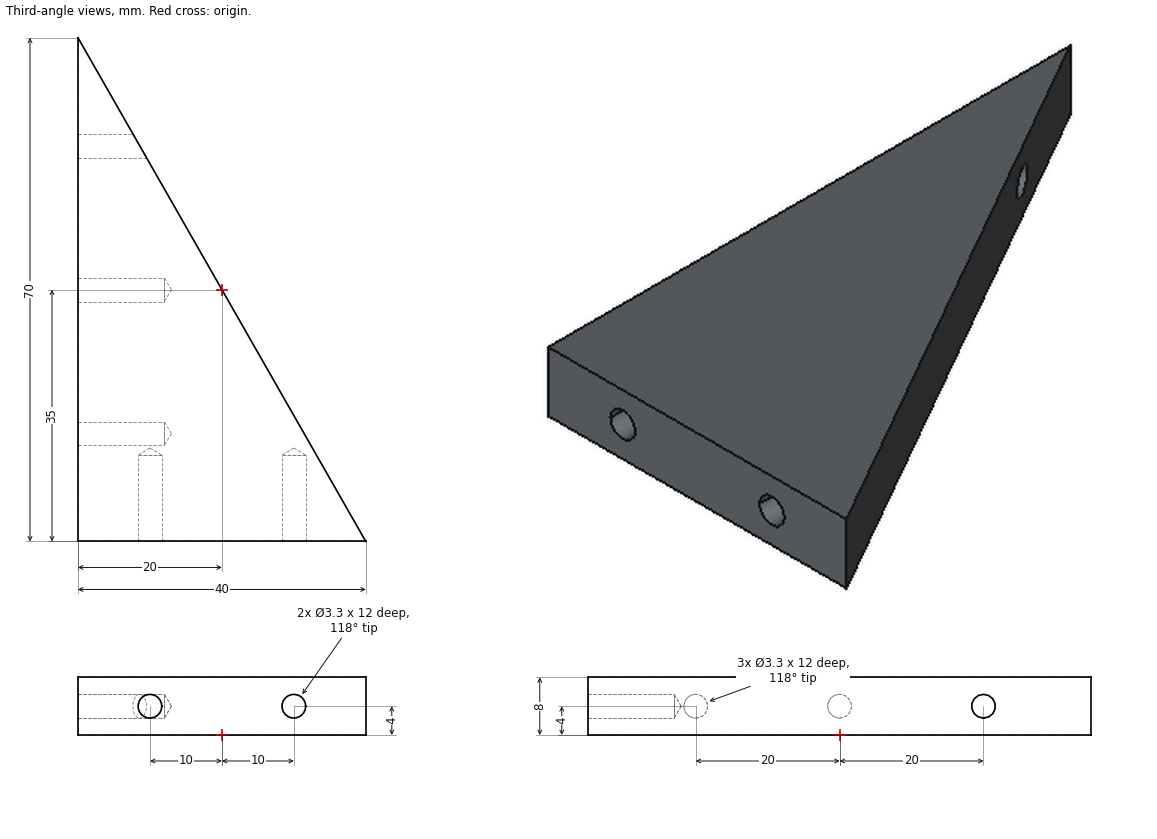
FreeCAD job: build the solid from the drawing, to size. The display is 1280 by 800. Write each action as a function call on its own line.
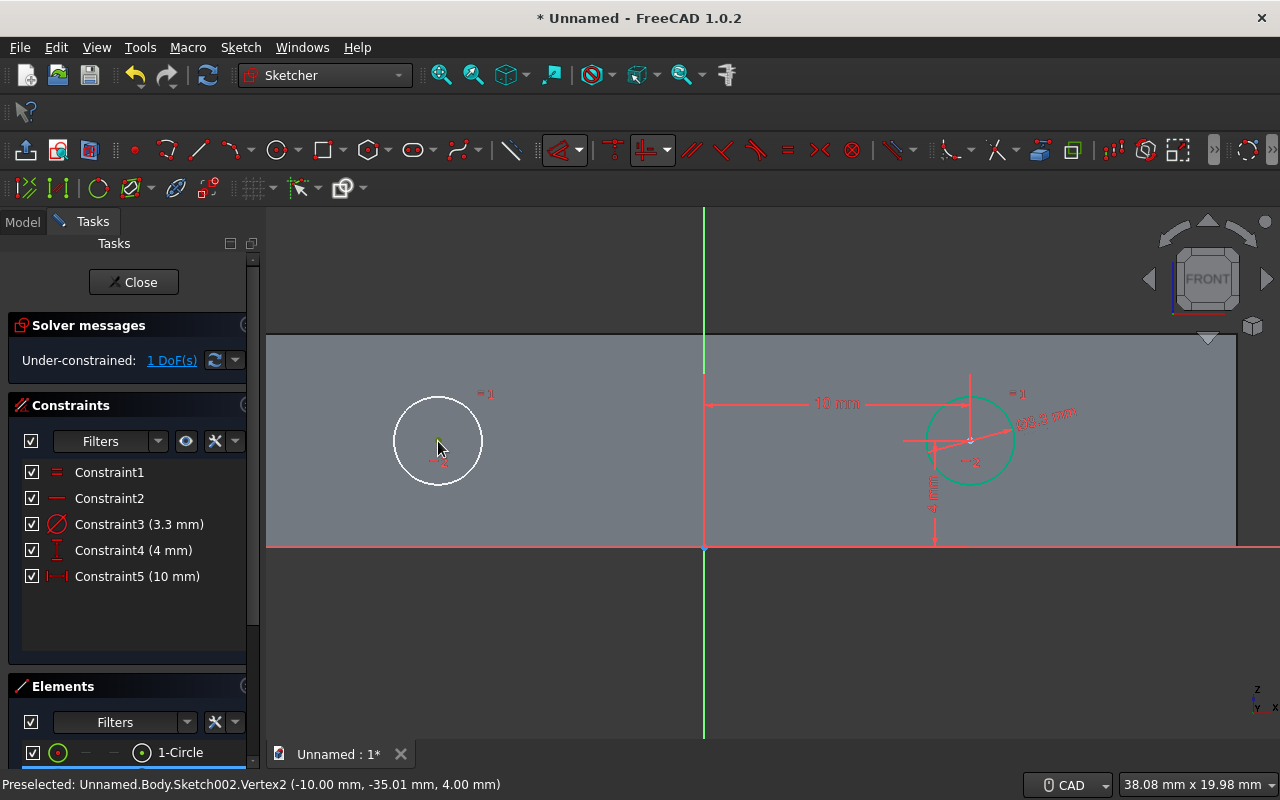
click(582, 150)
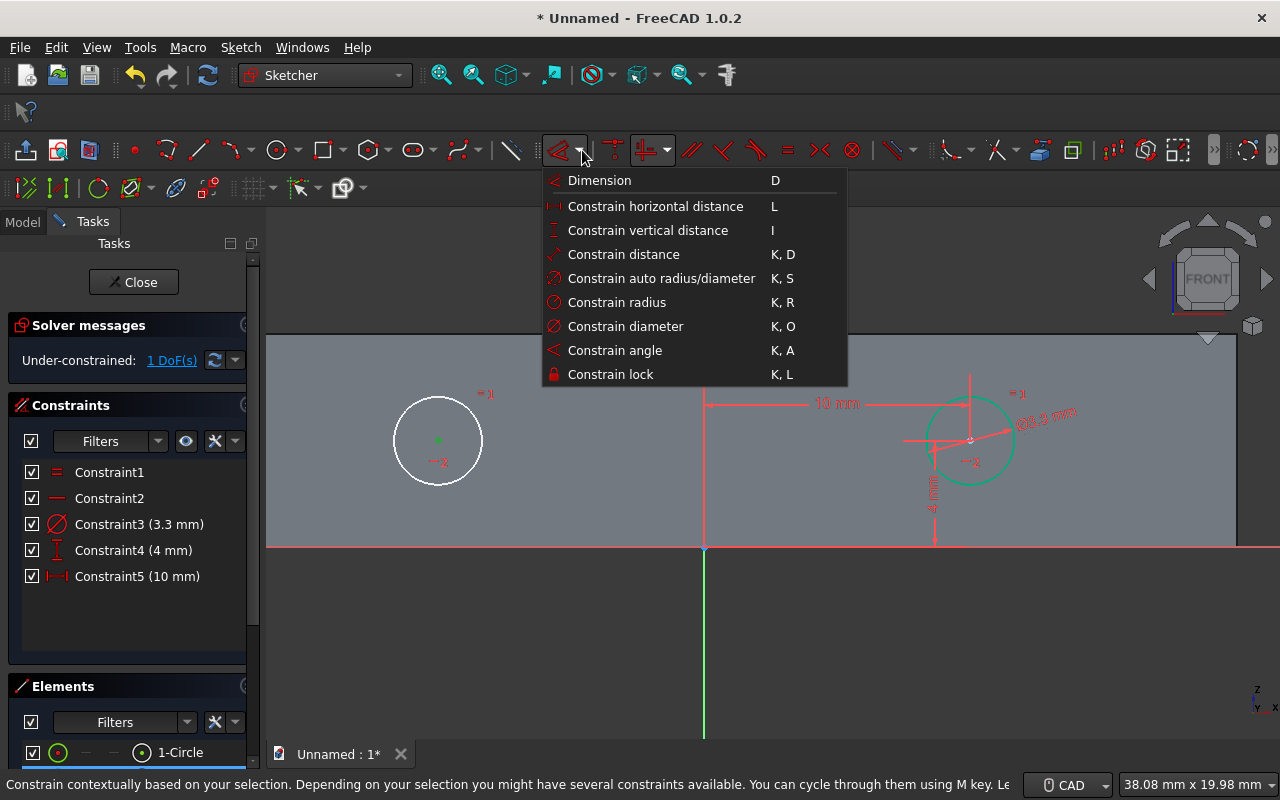
click(695, 206)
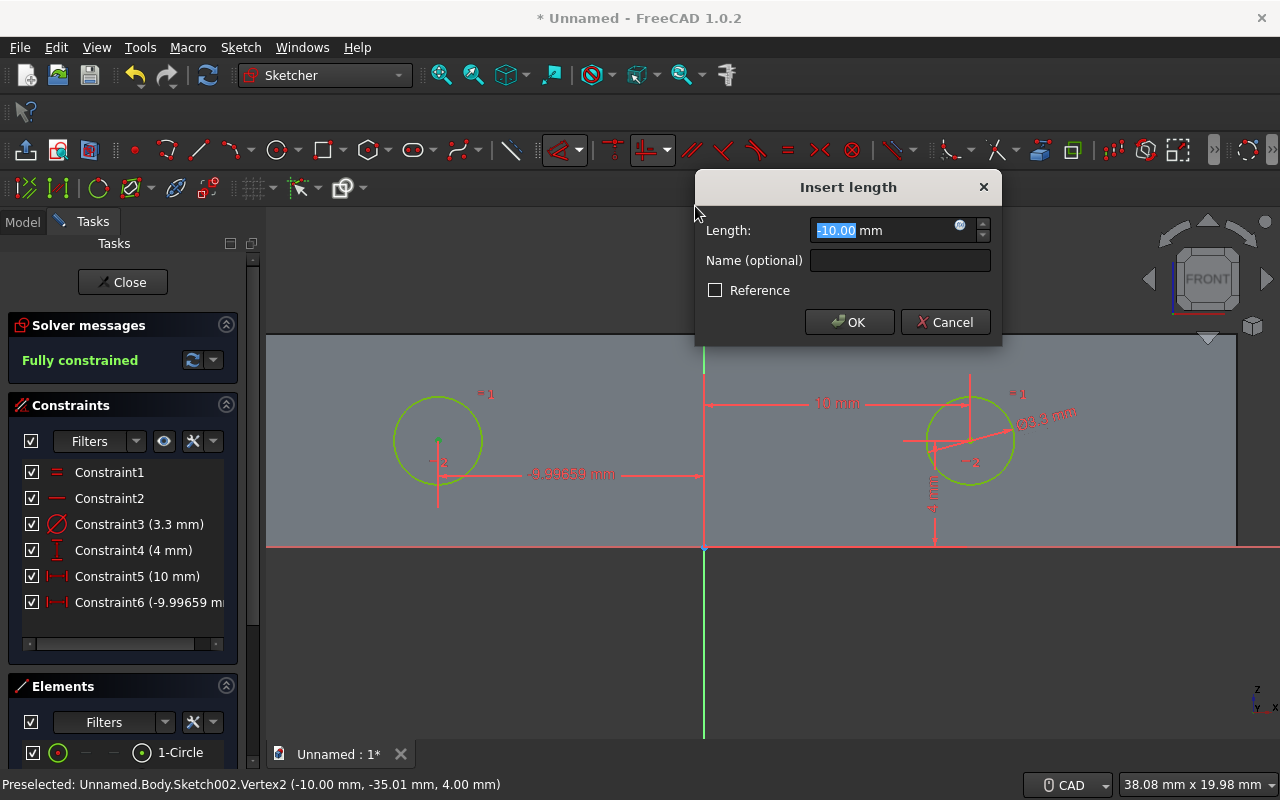
text(-10)
key(Return)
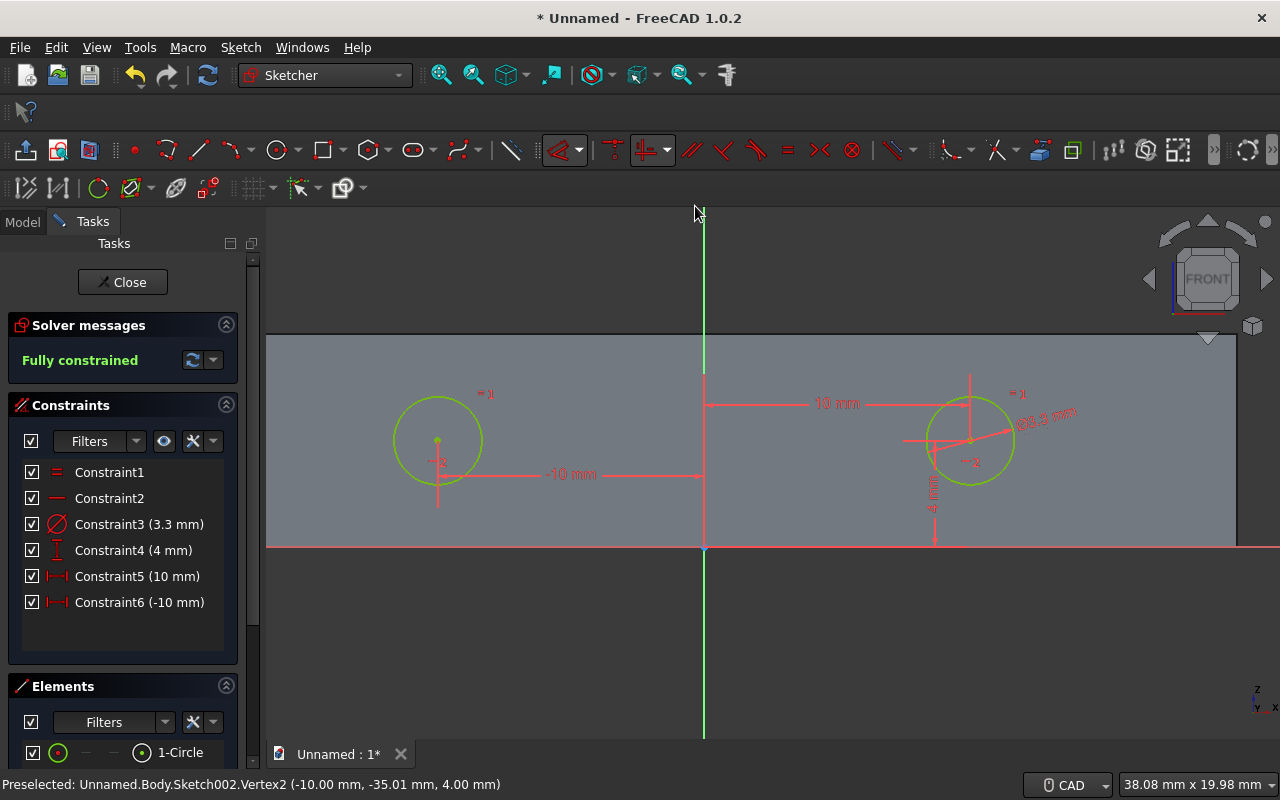
click(123, 282)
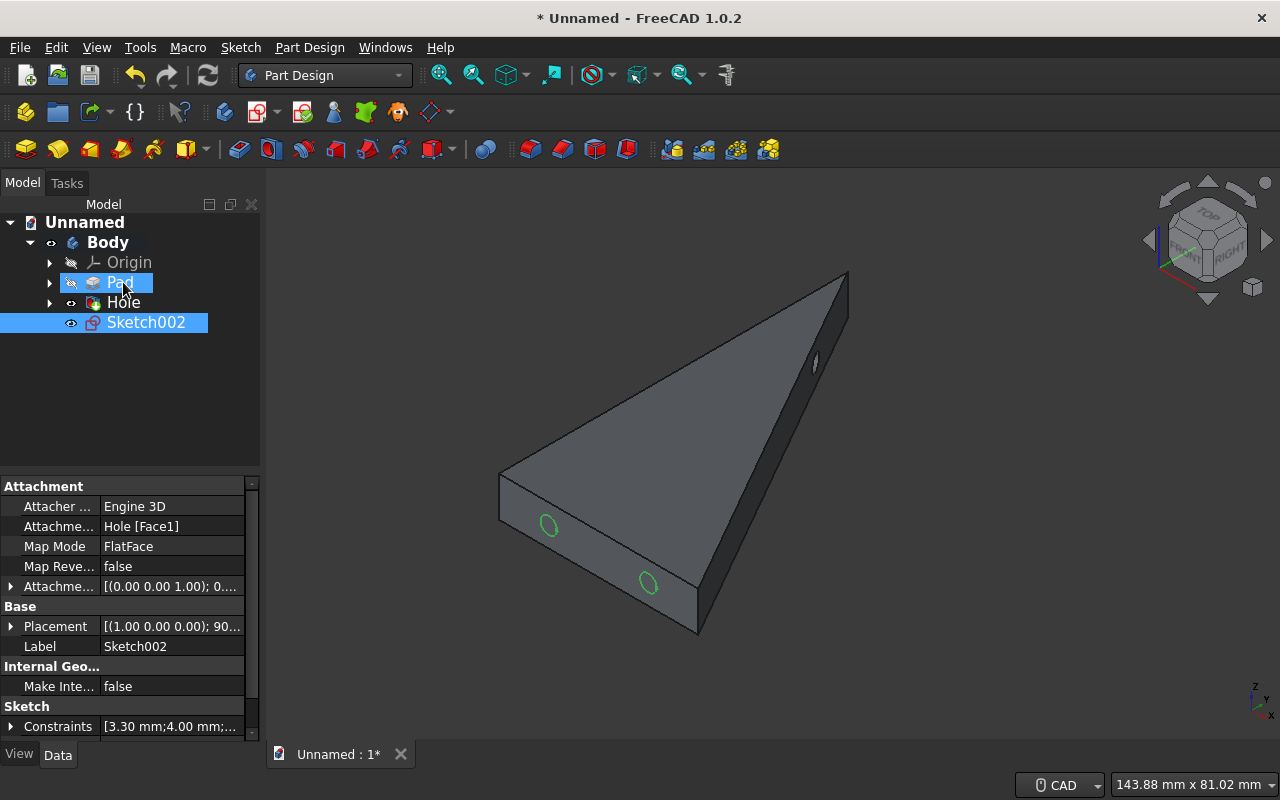
click(272, 150)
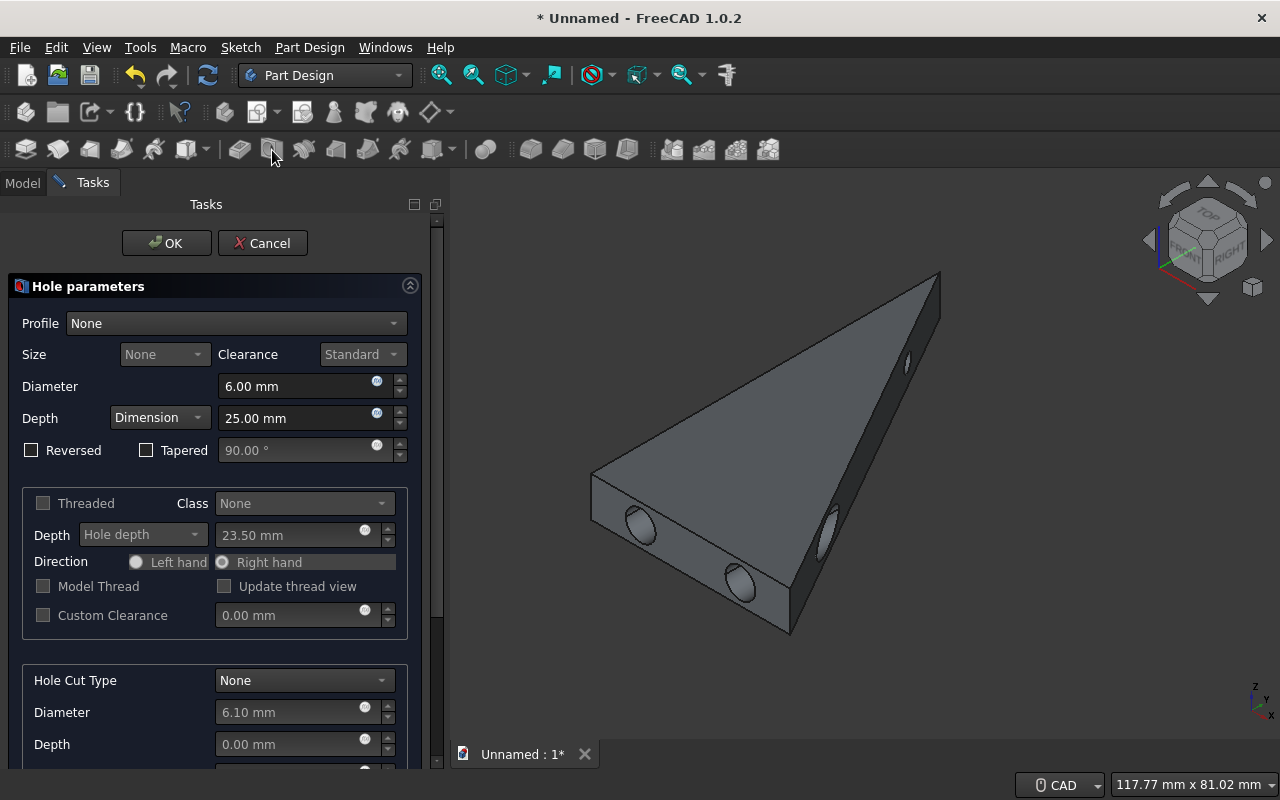
triple_click(305, 386)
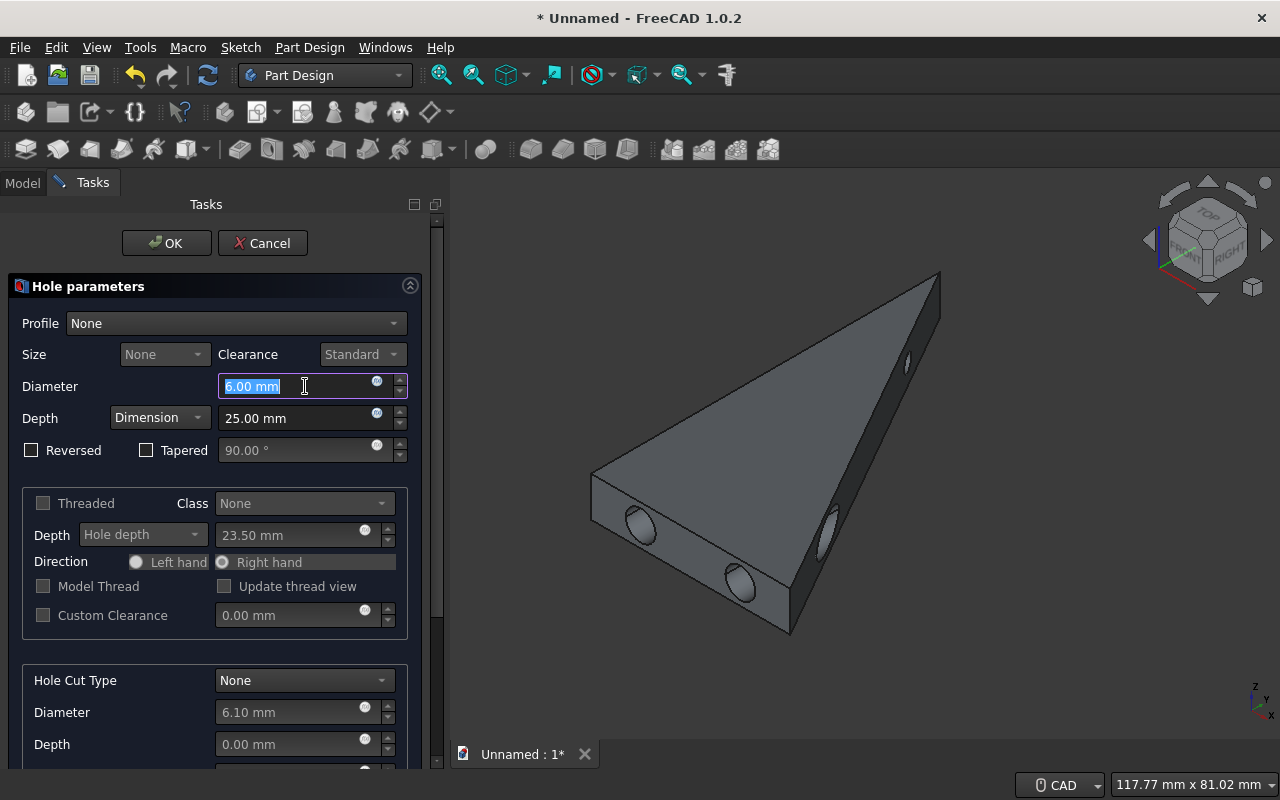
text(3.3)
key(Tab)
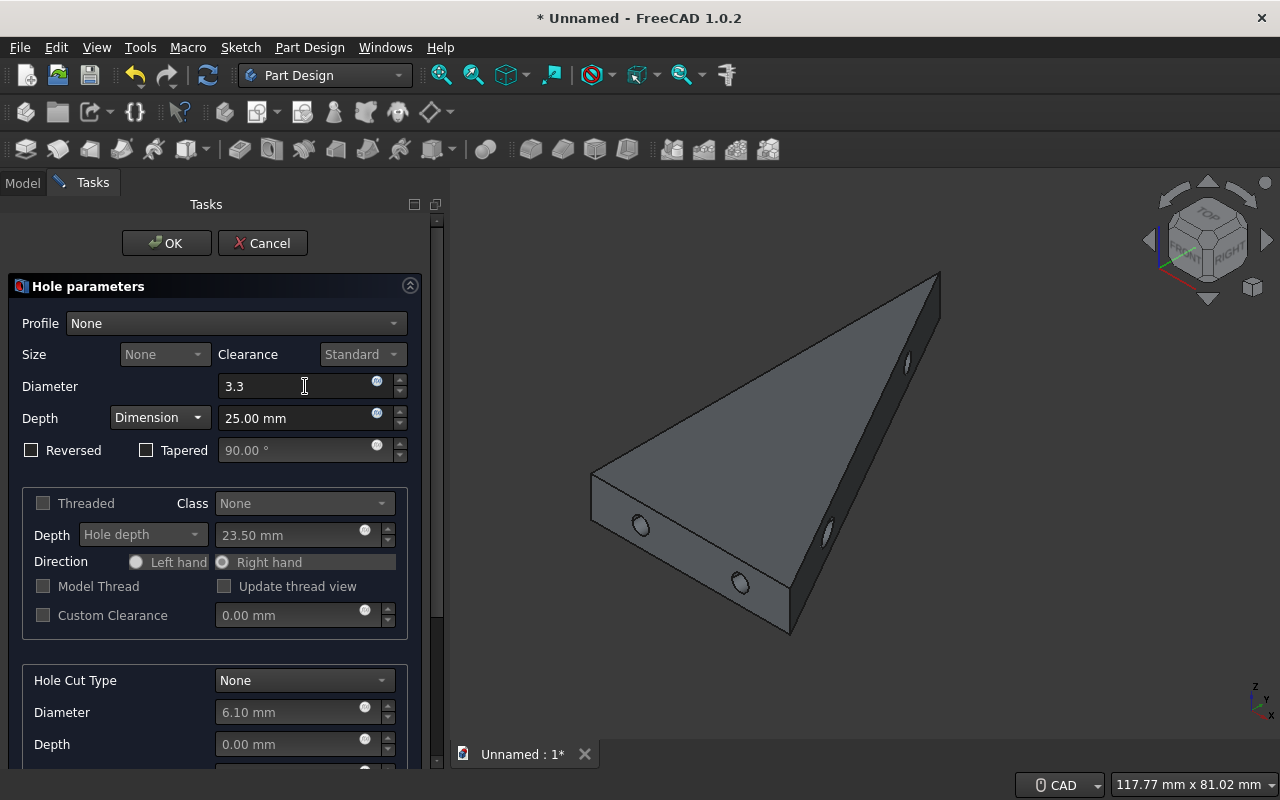
triple_click(305, 418)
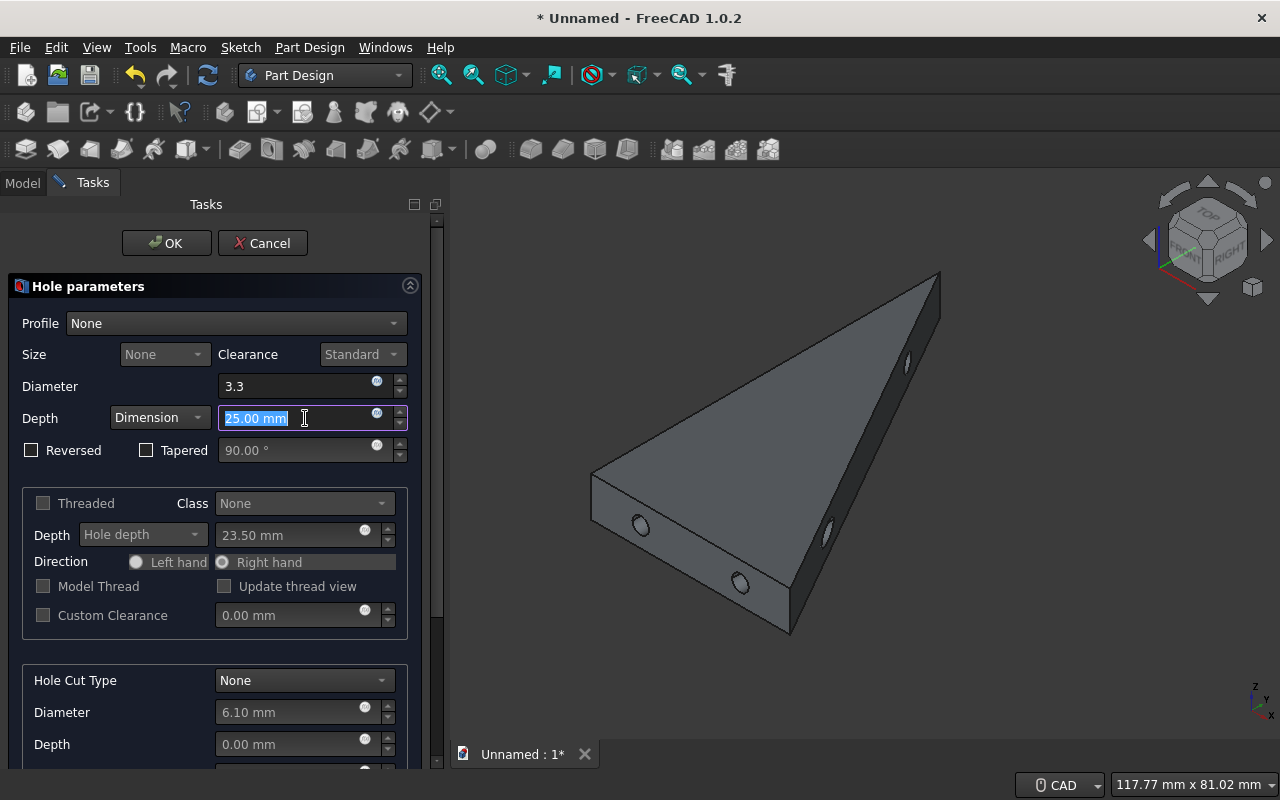
text(12)
key(Tab)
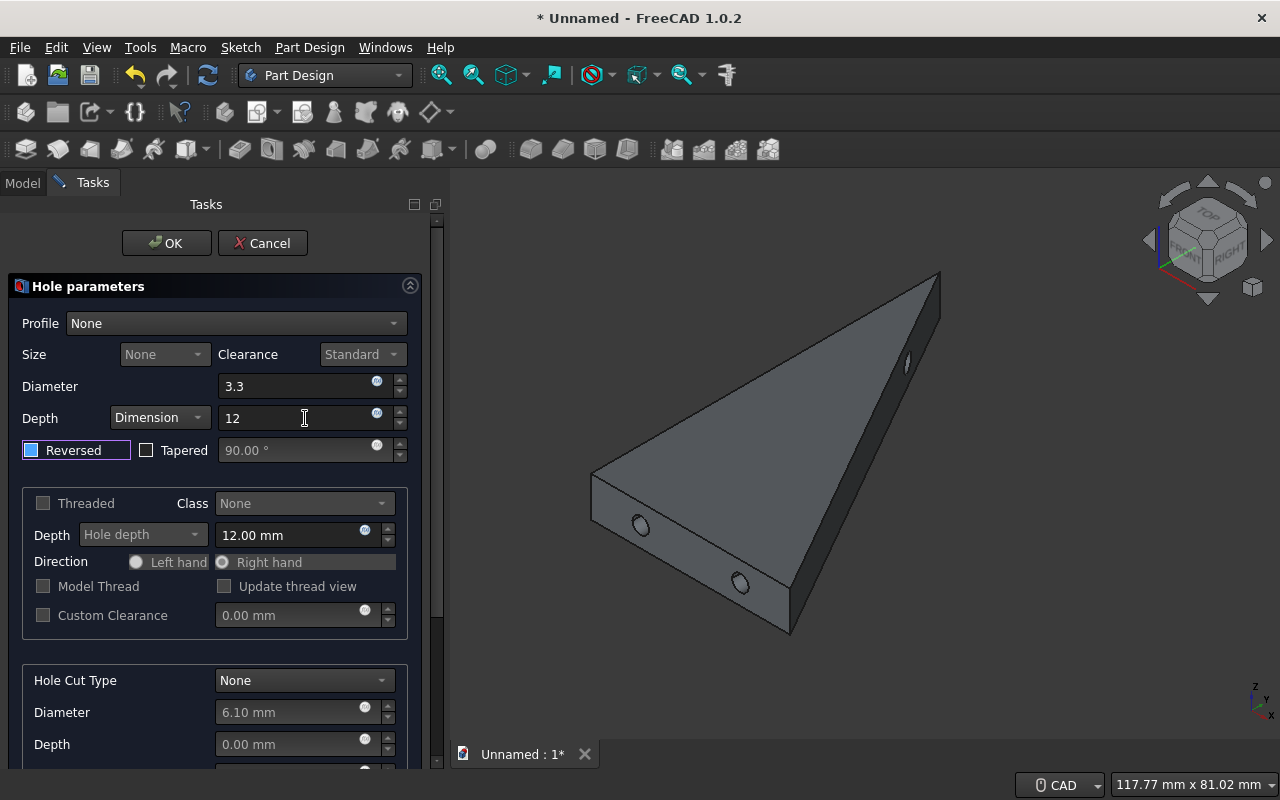
click(167, 243)